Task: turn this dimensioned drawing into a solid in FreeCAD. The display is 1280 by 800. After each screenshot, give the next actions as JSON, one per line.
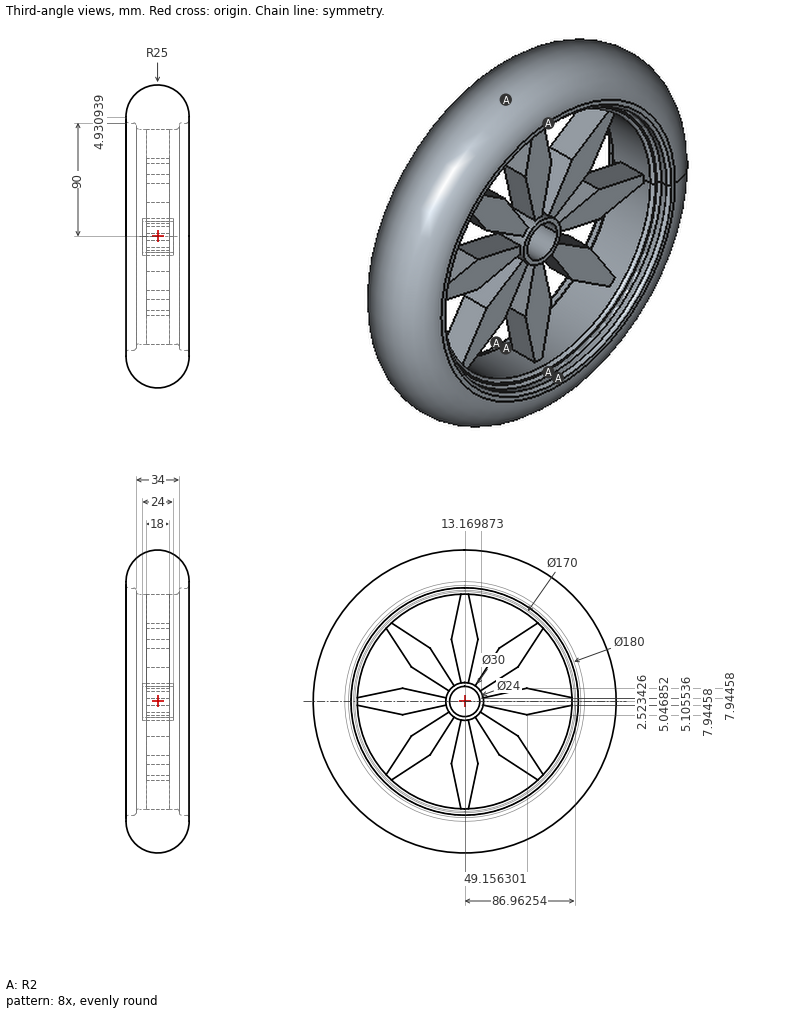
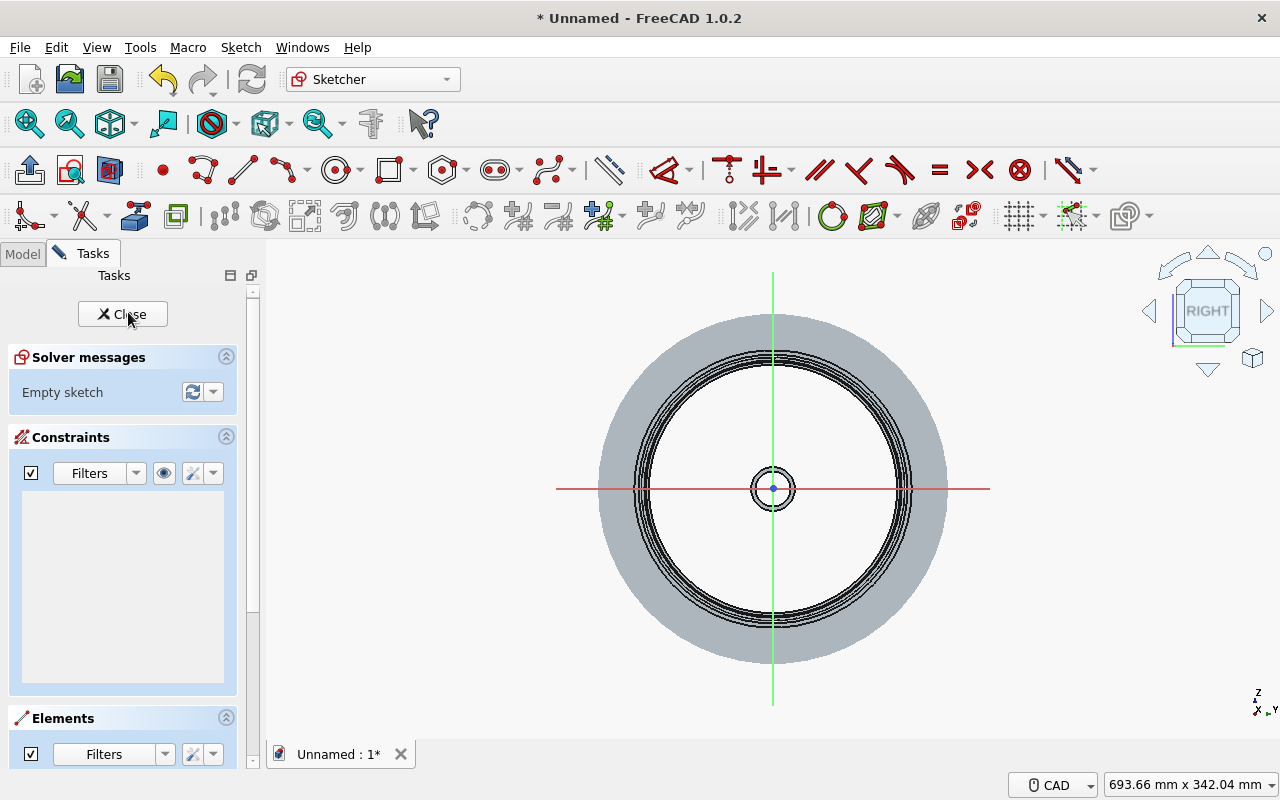
{"action": "scroll", "coordinate": [870, 489], "scroll_direction": "up", "scroll_amount": 8}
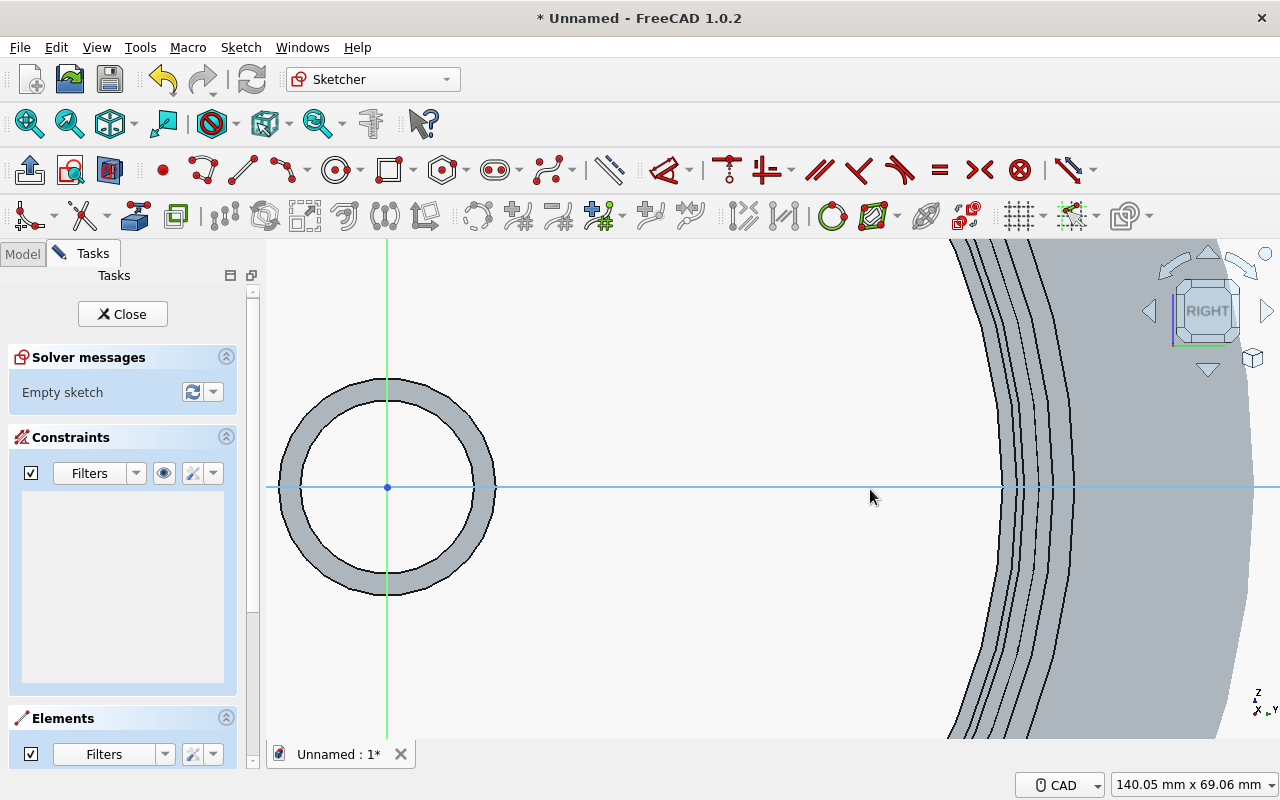
{"action": "left_click", "coordinate": [204, 170]}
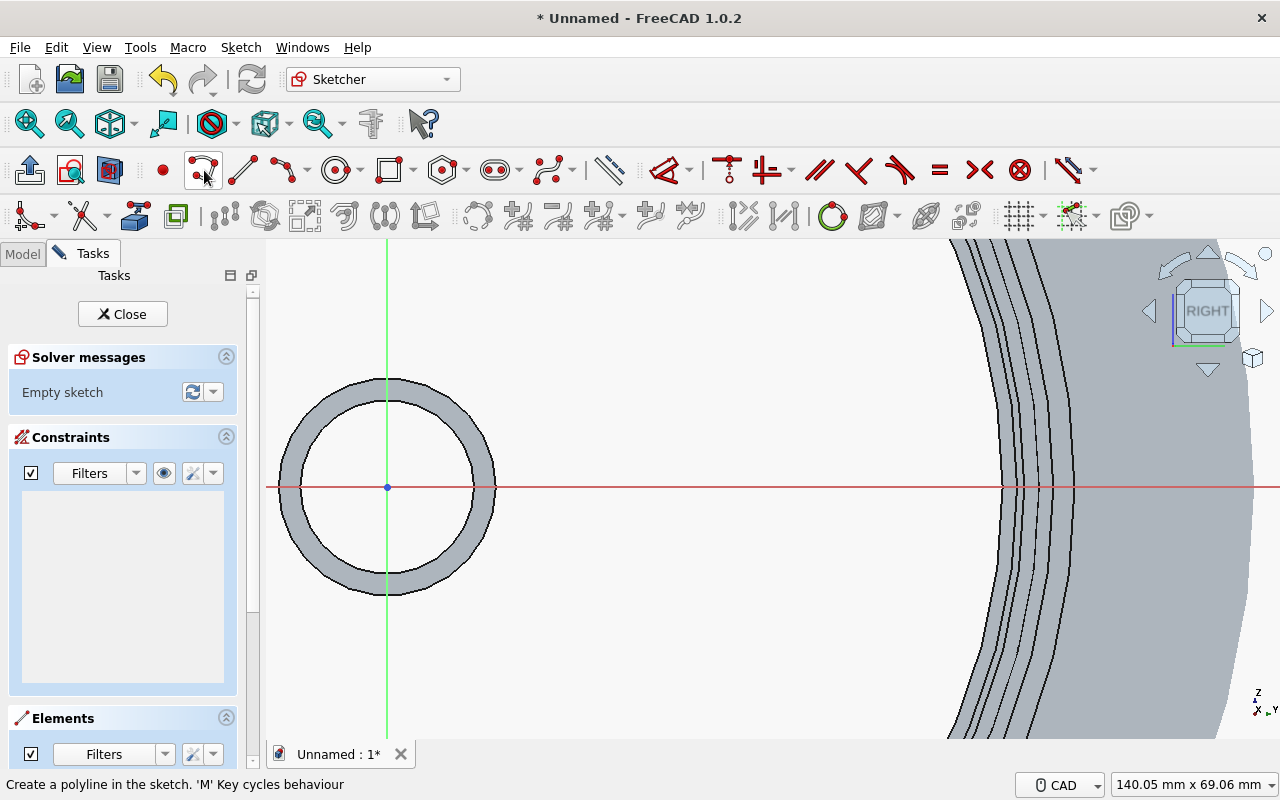
{"action": "left_click", "coordinate": [483, 469]}
{"action": "left_click", "coordinate": [483, 505]}
{"action": "left_click", "coordinate": [743, 563]}
{"action": "left_click", "coordinate": [1017, 506]}
{"action": "left_click", "coordinate": [1017, 469]}
{"action": "left_click", "coordinate": [743, 411]}
{"action": "left_click", "coordinate": [483, 470]}
{"action": "key", "text": "Escape"}
{"action": "key", "text": "Escape"}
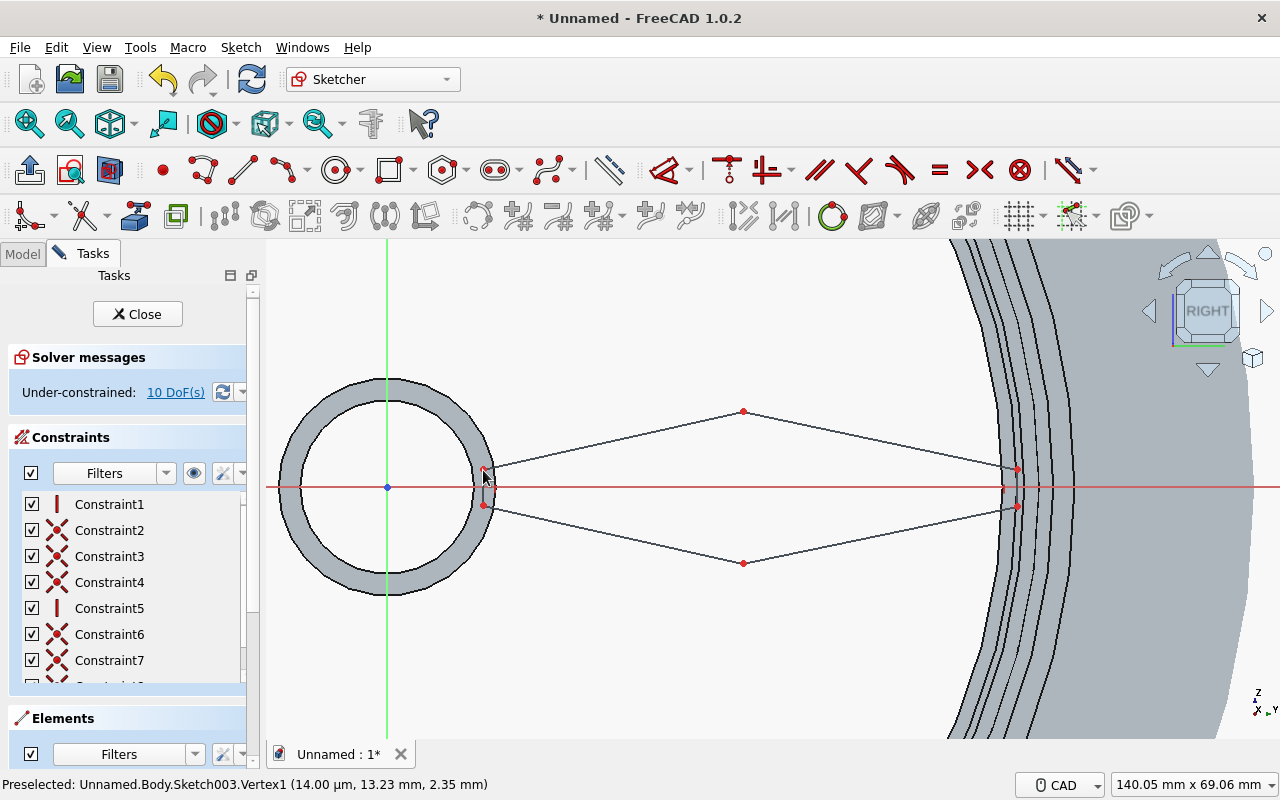
{"action": "left_click", "coordinate": [743, 564]}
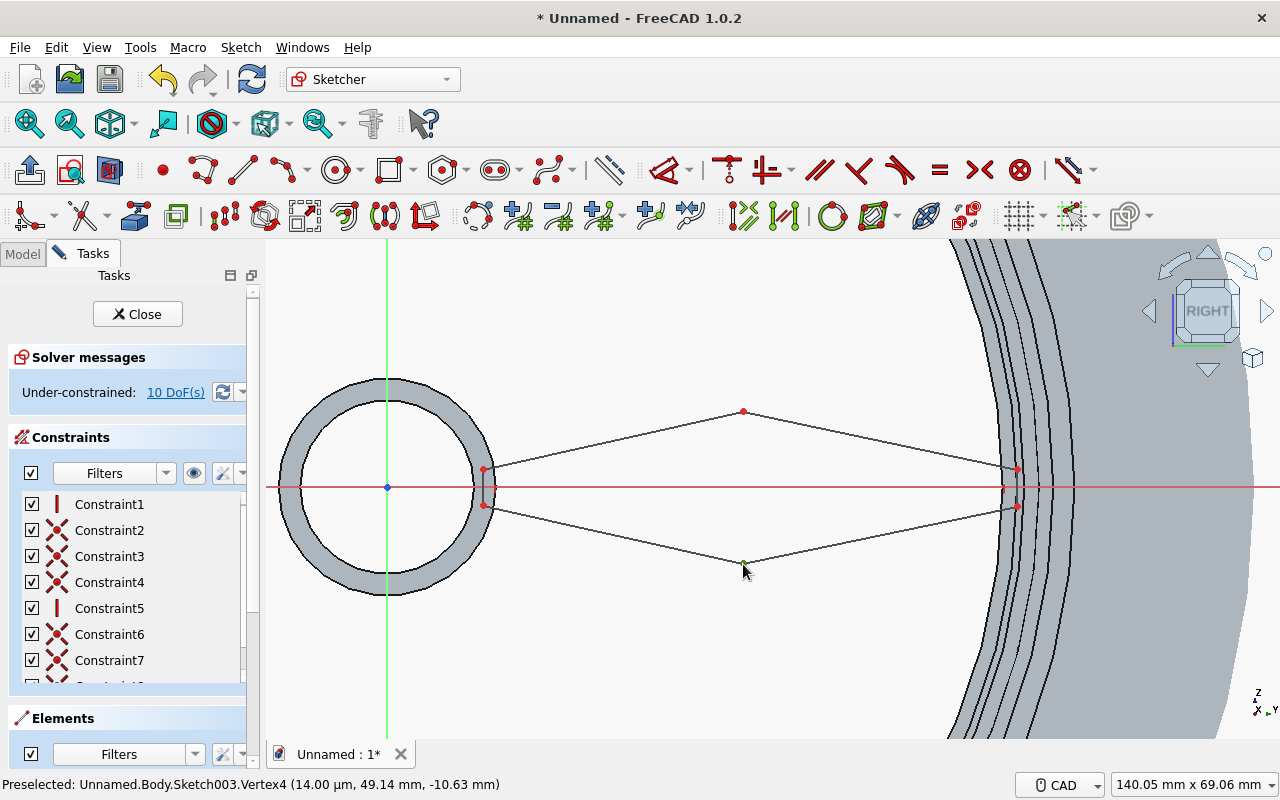
{"action": "left_click", "coordinate": [743, 412]}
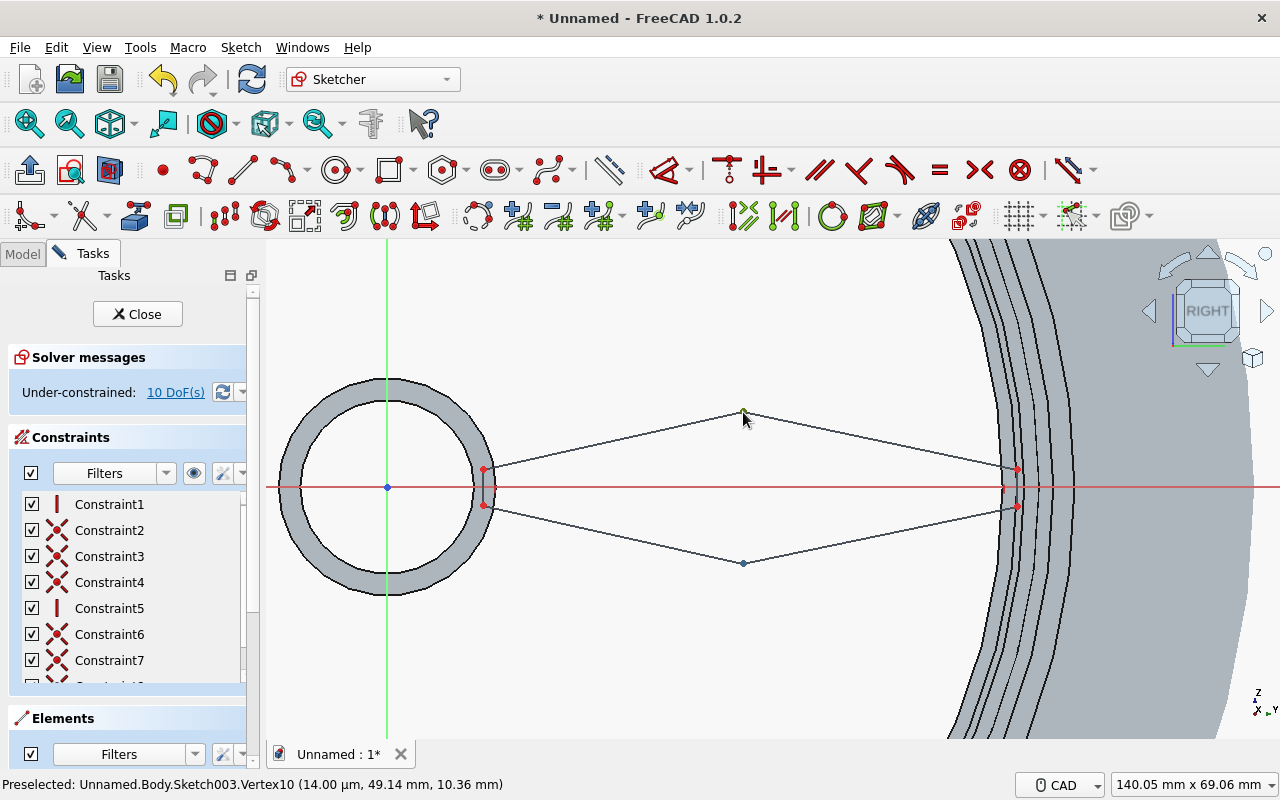
{"action": "left_click", "coordinate": [353, 487]}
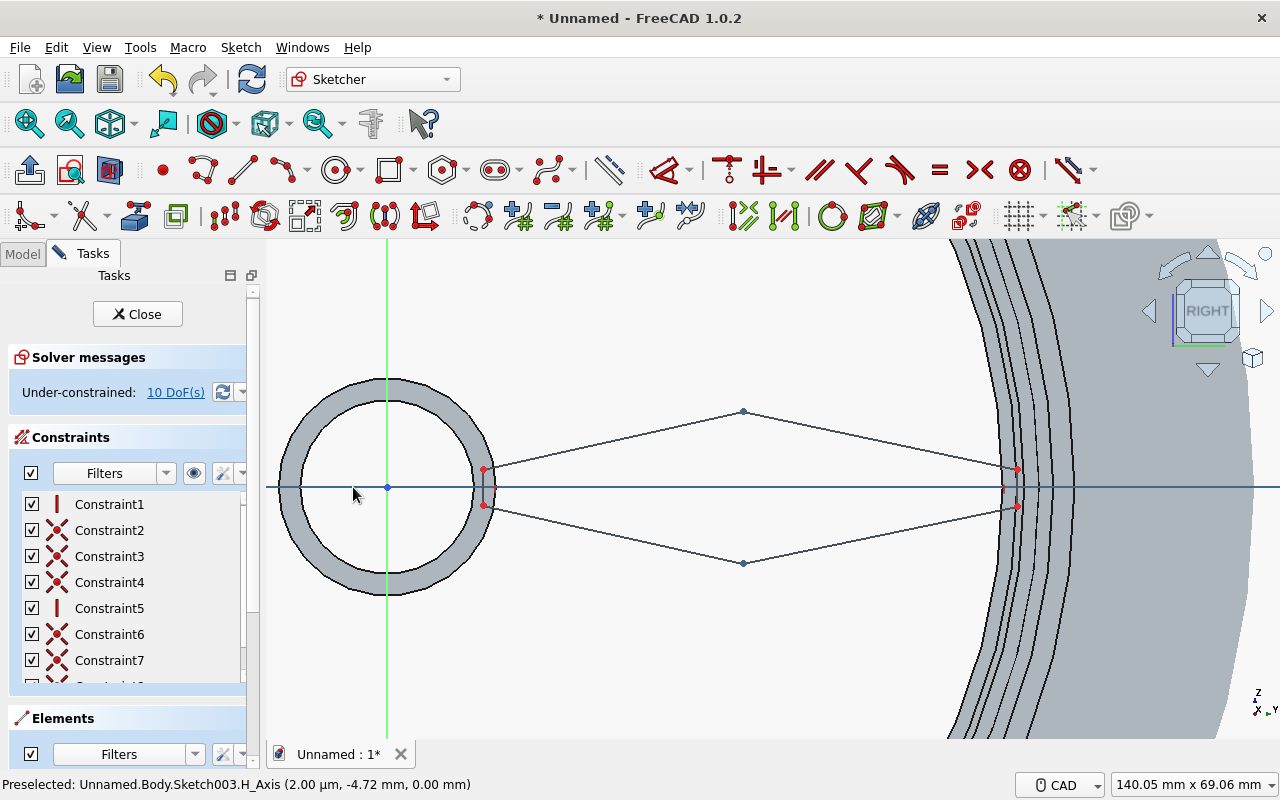
{"action": "left_click", "coordinate": [980, 170]}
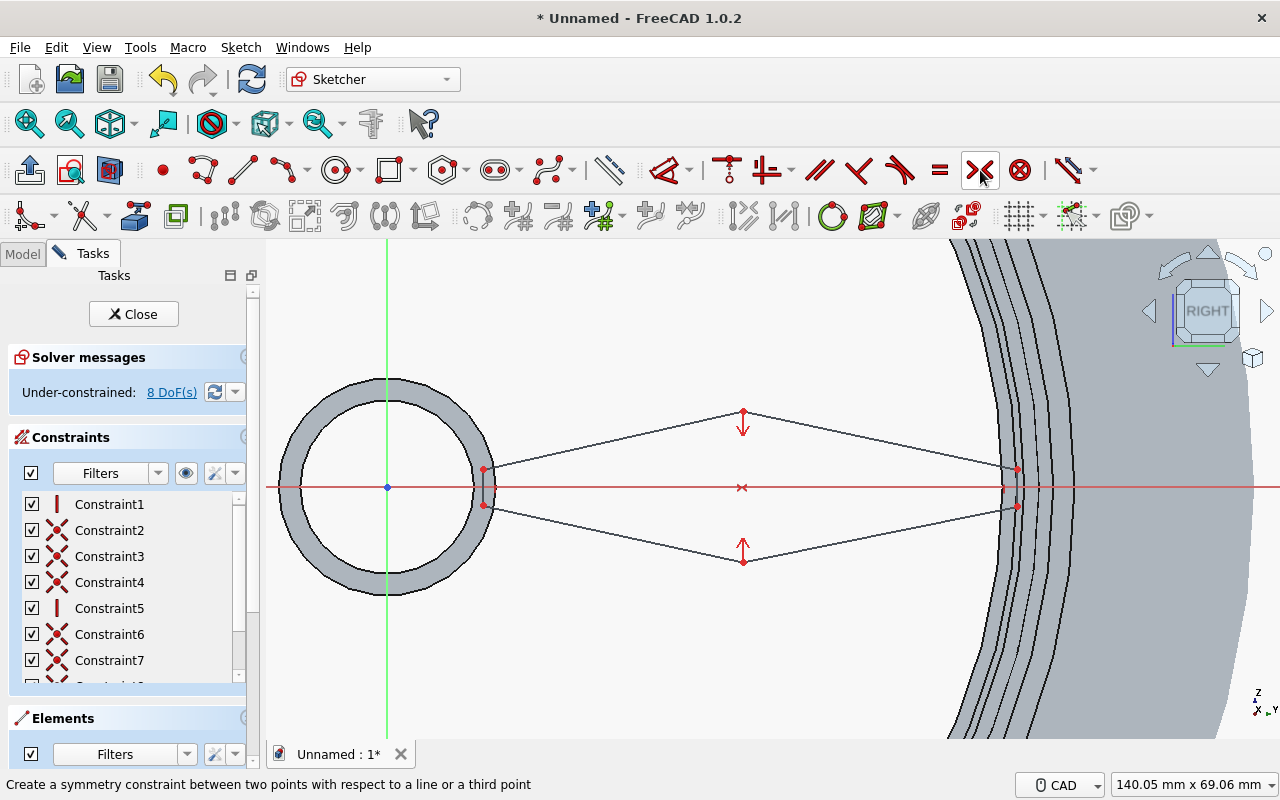
{"action": "key", "text": "d"}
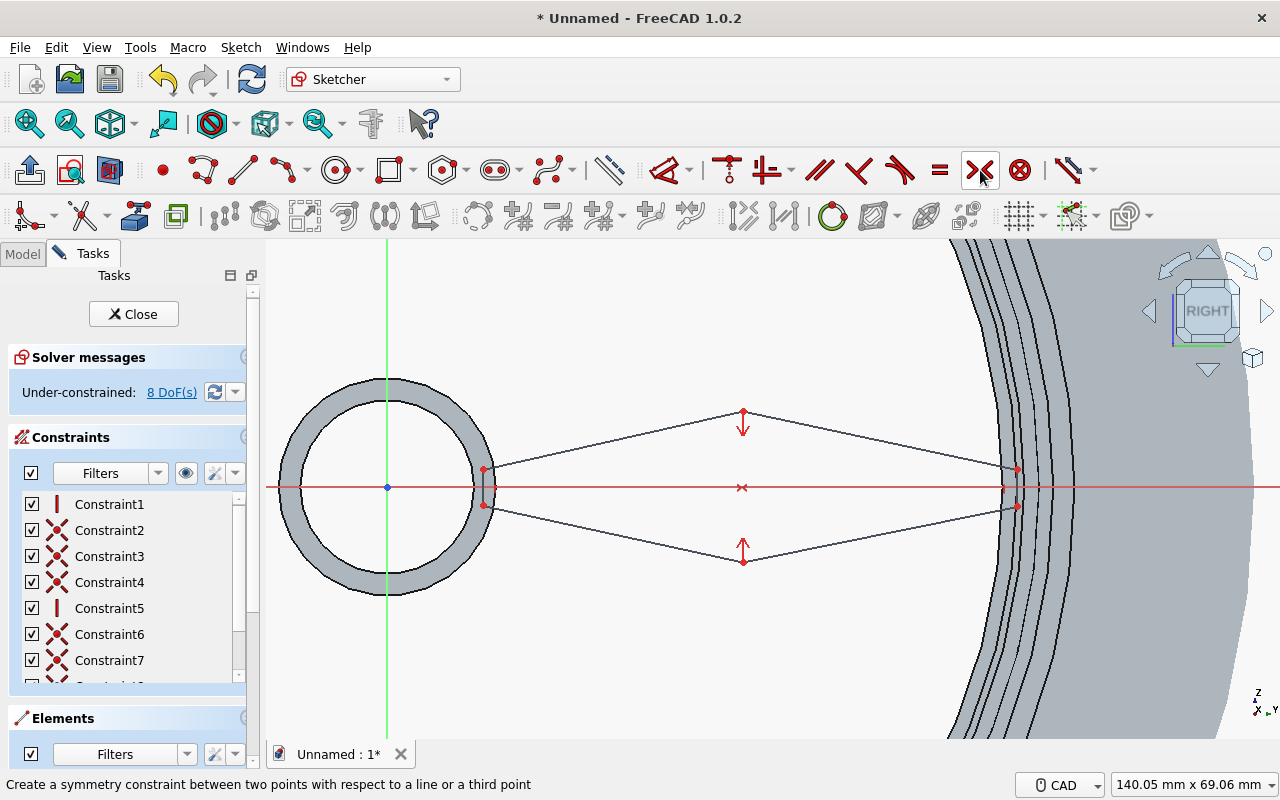
{"action": "left_click", "coordinate": [483, 484]}
{"action": "left_click", "coordinate": [449, 501]}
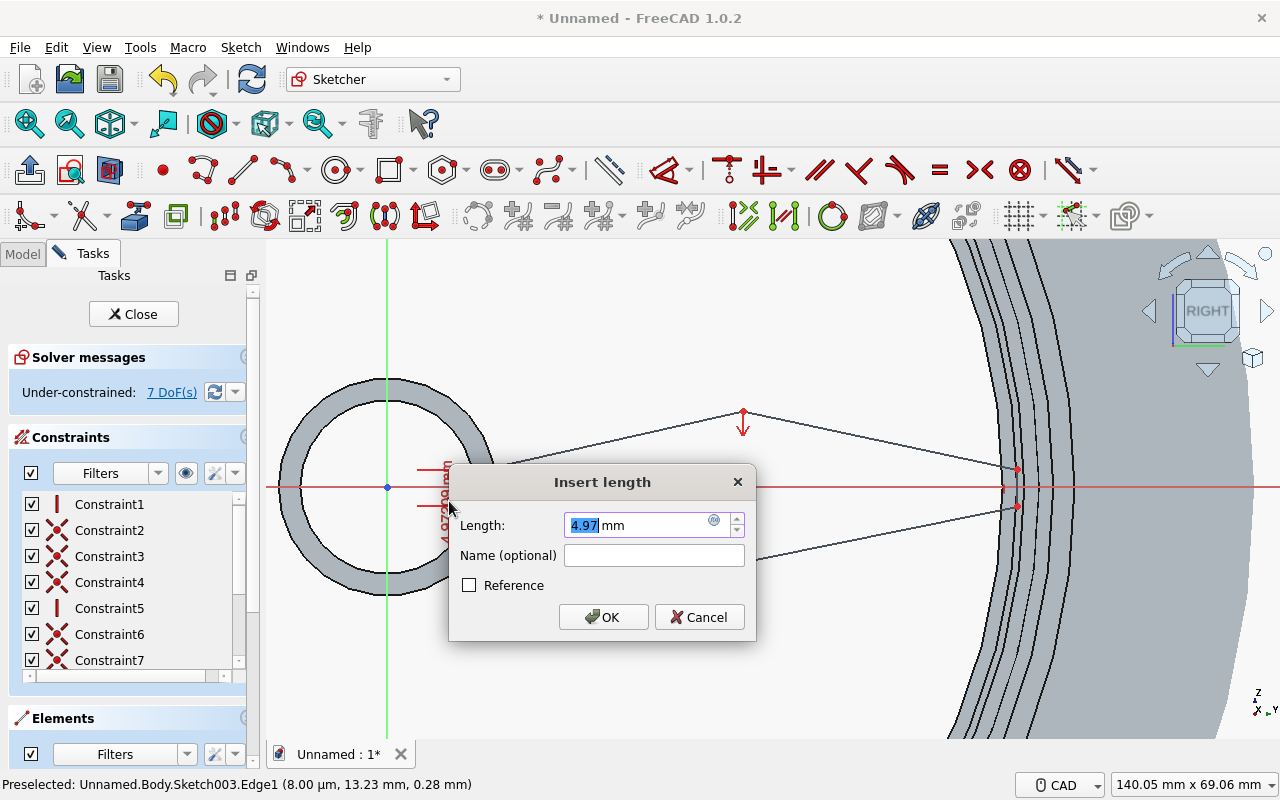
{"action": "type", "text": "5.046852"}
{"action": "key", "text": "Return"}